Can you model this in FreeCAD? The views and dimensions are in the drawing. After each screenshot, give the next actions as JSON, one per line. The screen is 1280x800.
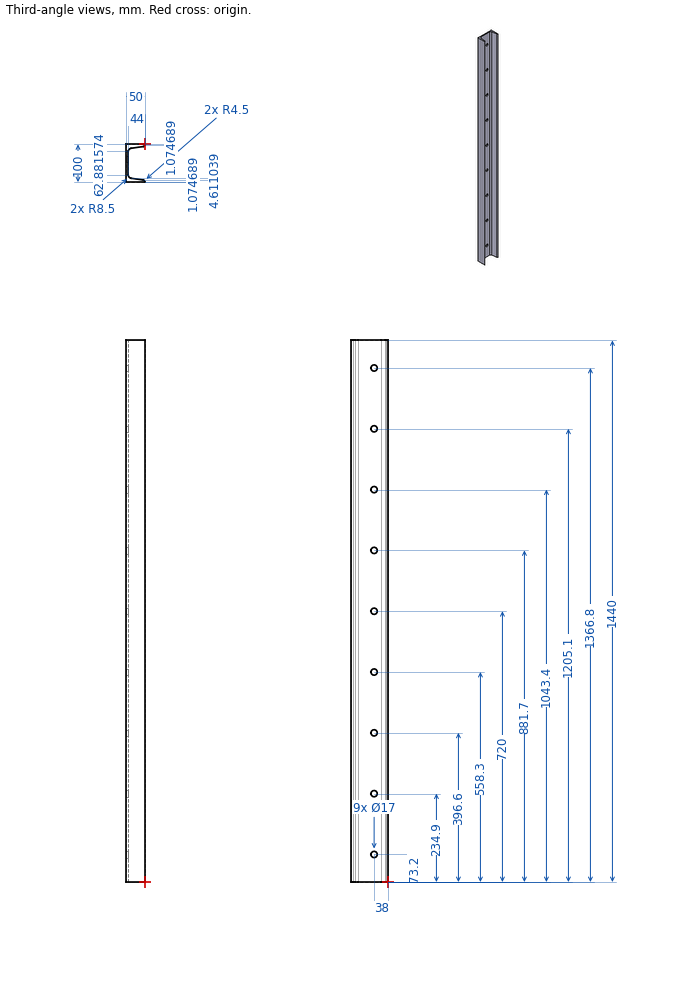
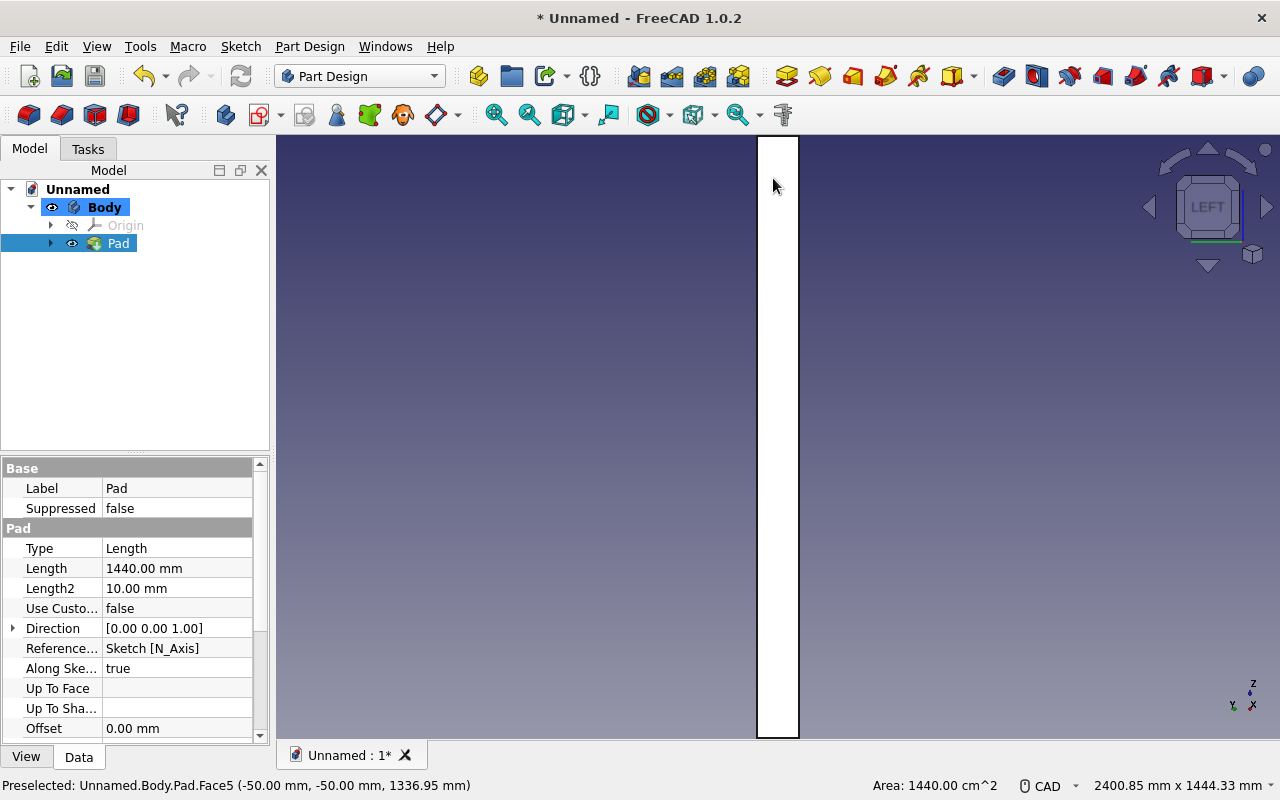
{"action": "left_click", "coordinate": [258, 116]}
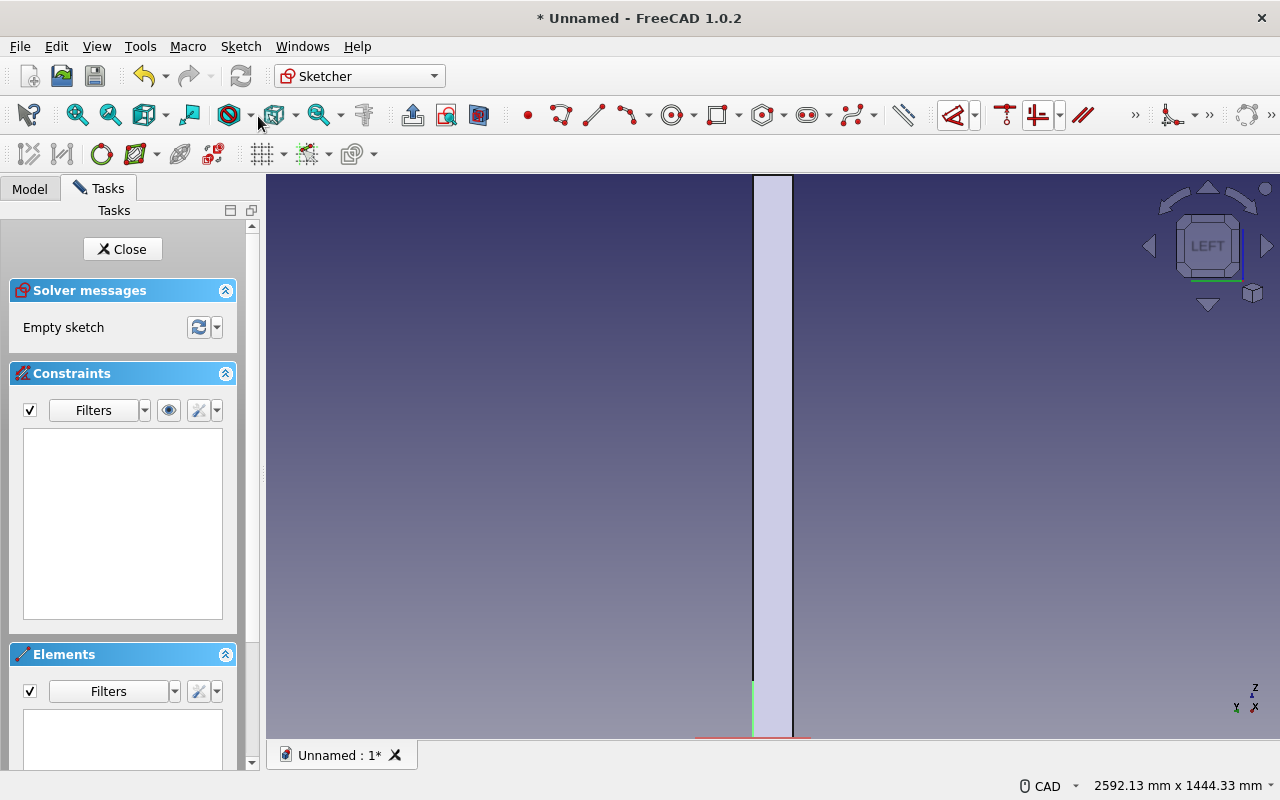
{"action": "scroll", "coordinate": [586, 431], "scroll_direction": "down", "scroll_amount": 2}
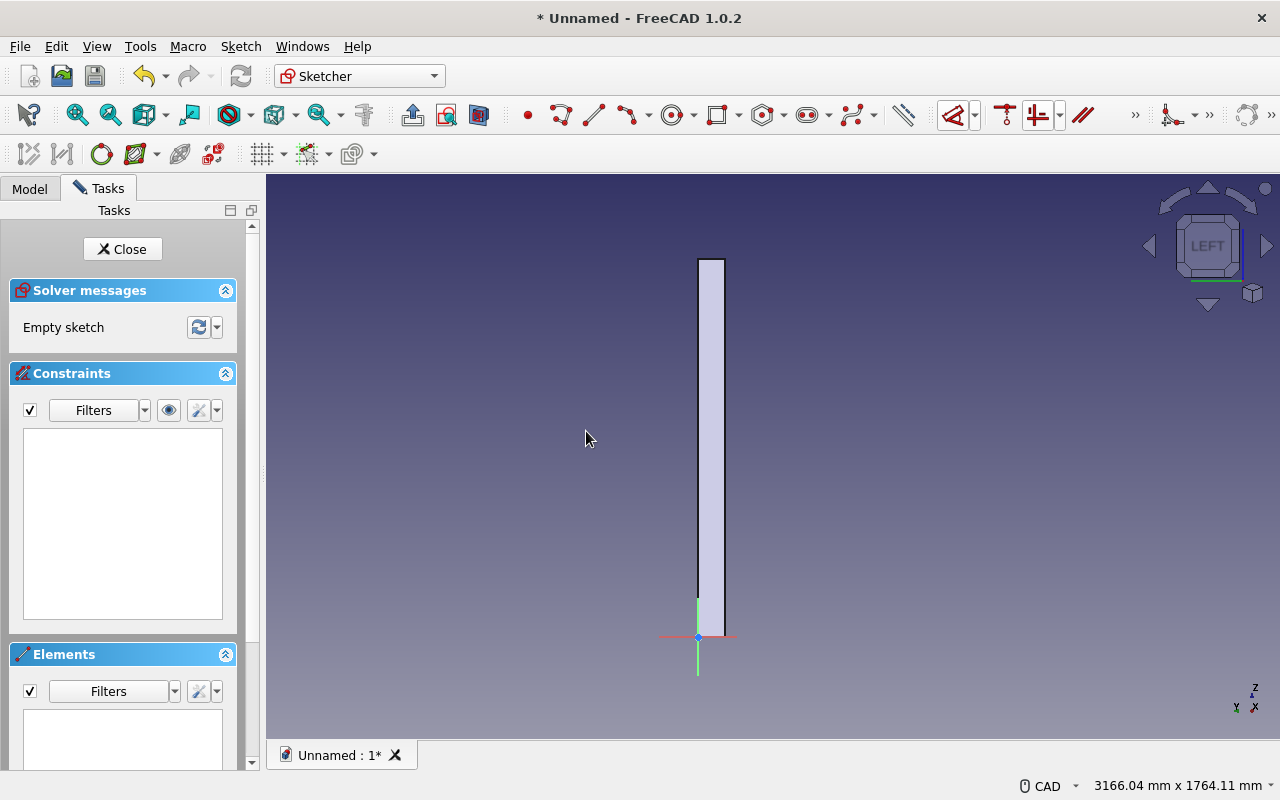
{"action": "left_click", "coordinate": [672, 116]}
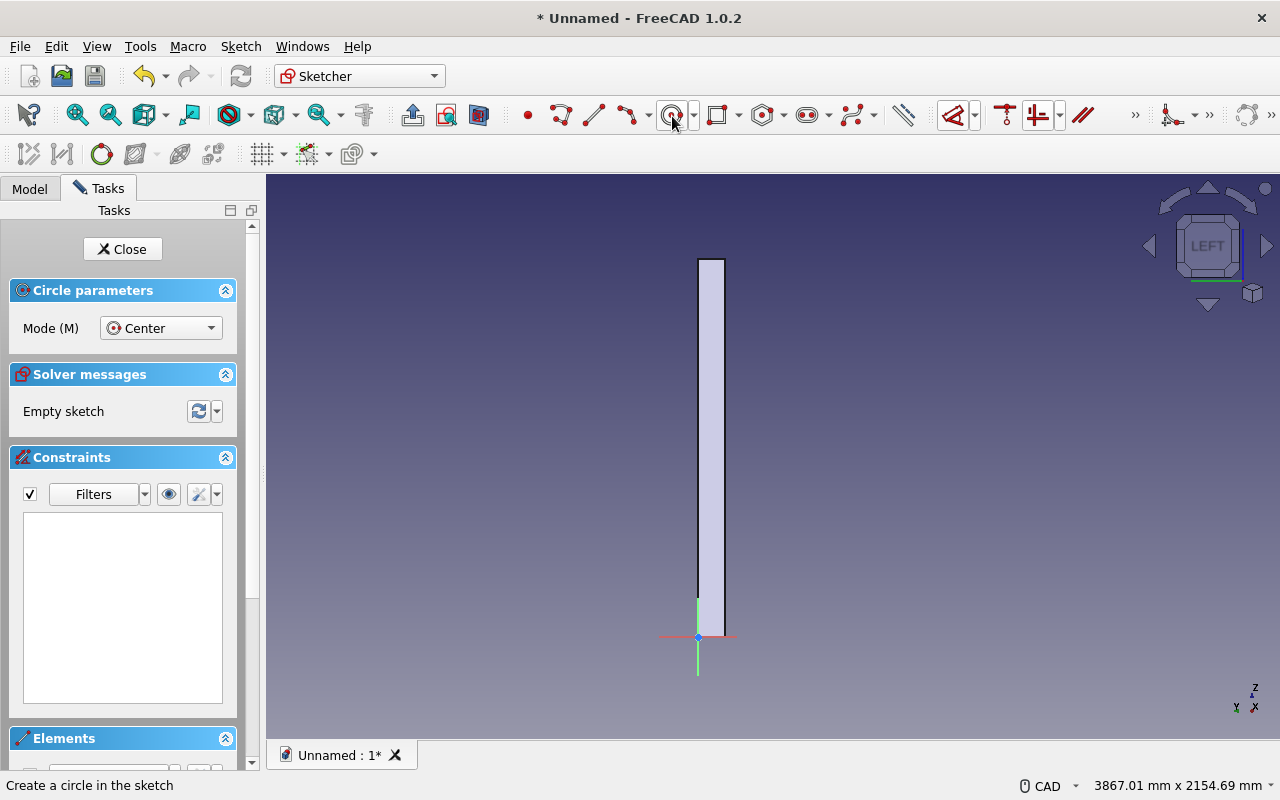
{"action": "scroll", "coordinate": [708, 618], "scroll_direction": "up", "scroll_amount": 12}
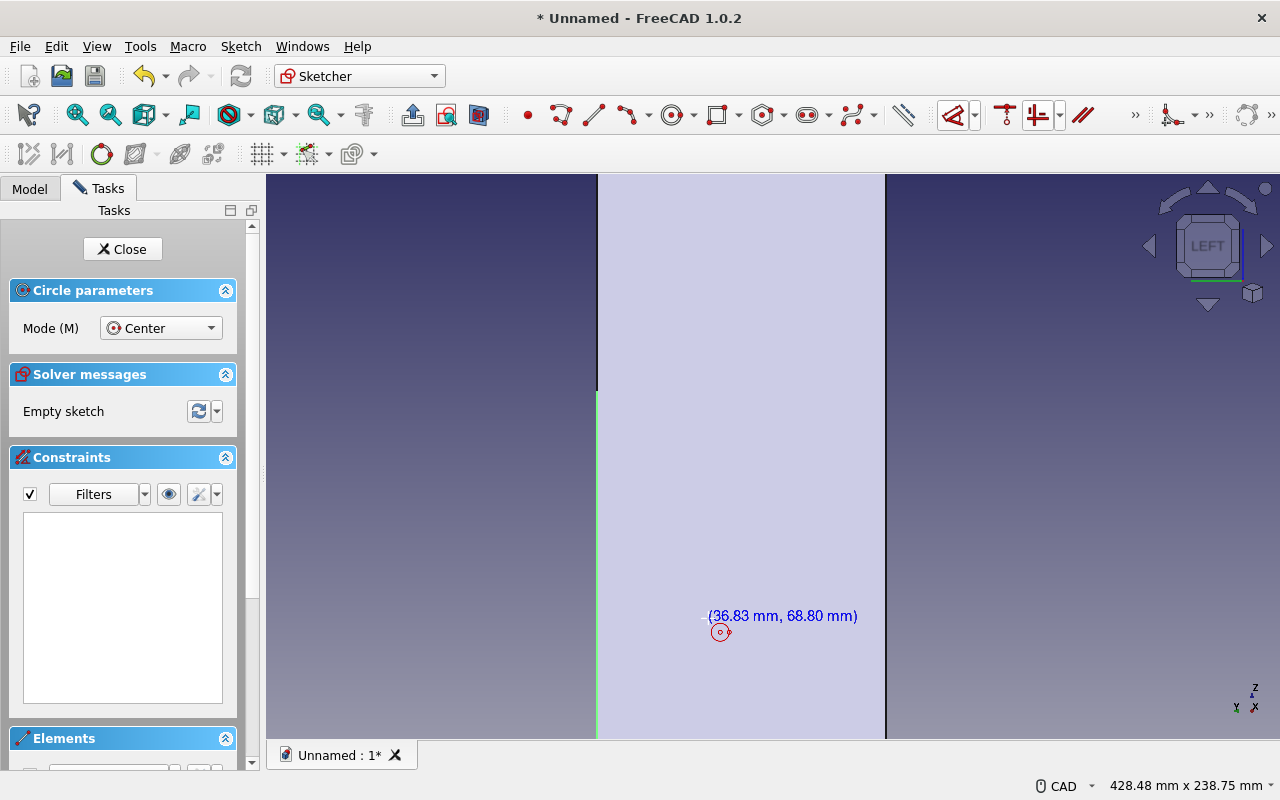
{"action": "scroll", "coordinate": [709, 619], "scroll_direction": "down", "scroll_amount": 12}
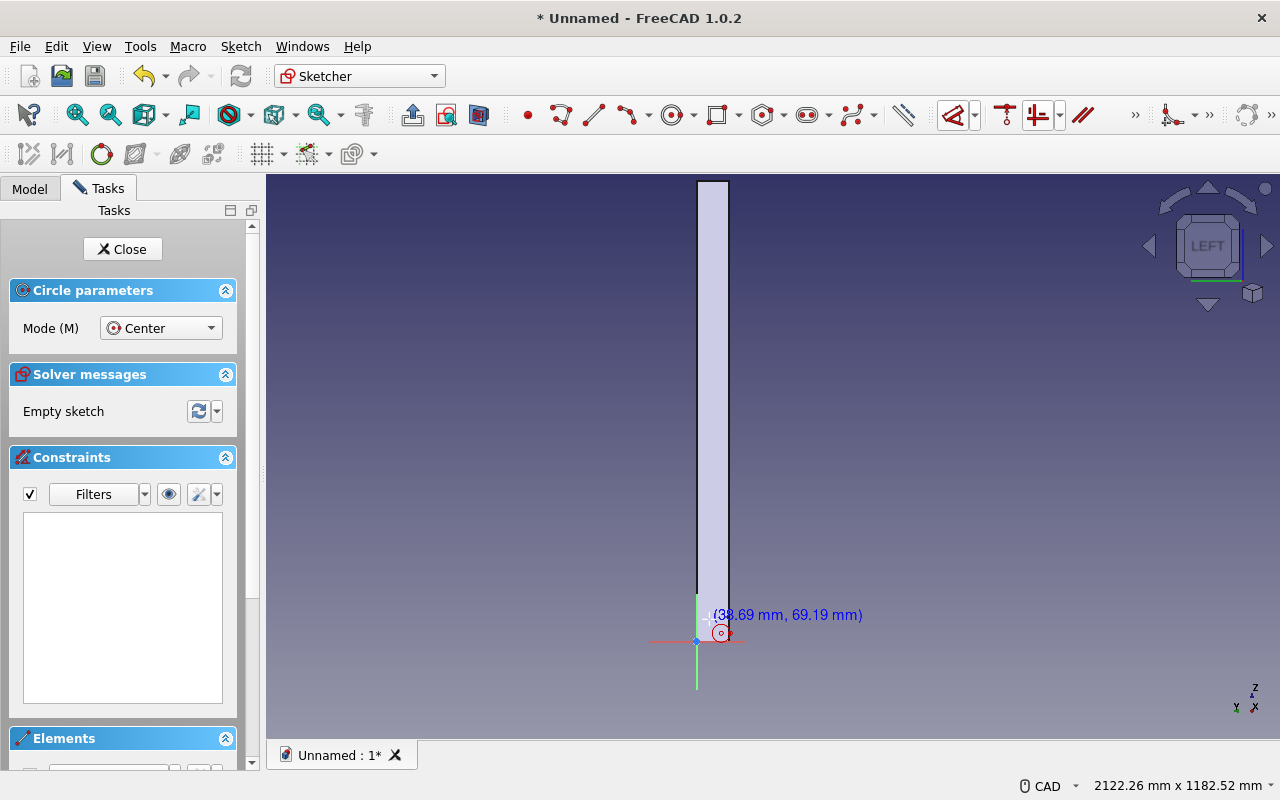
{"action": "scroll", "coordinate": [709, 619], "scroll_direction": "up", "scroll_amount": 3}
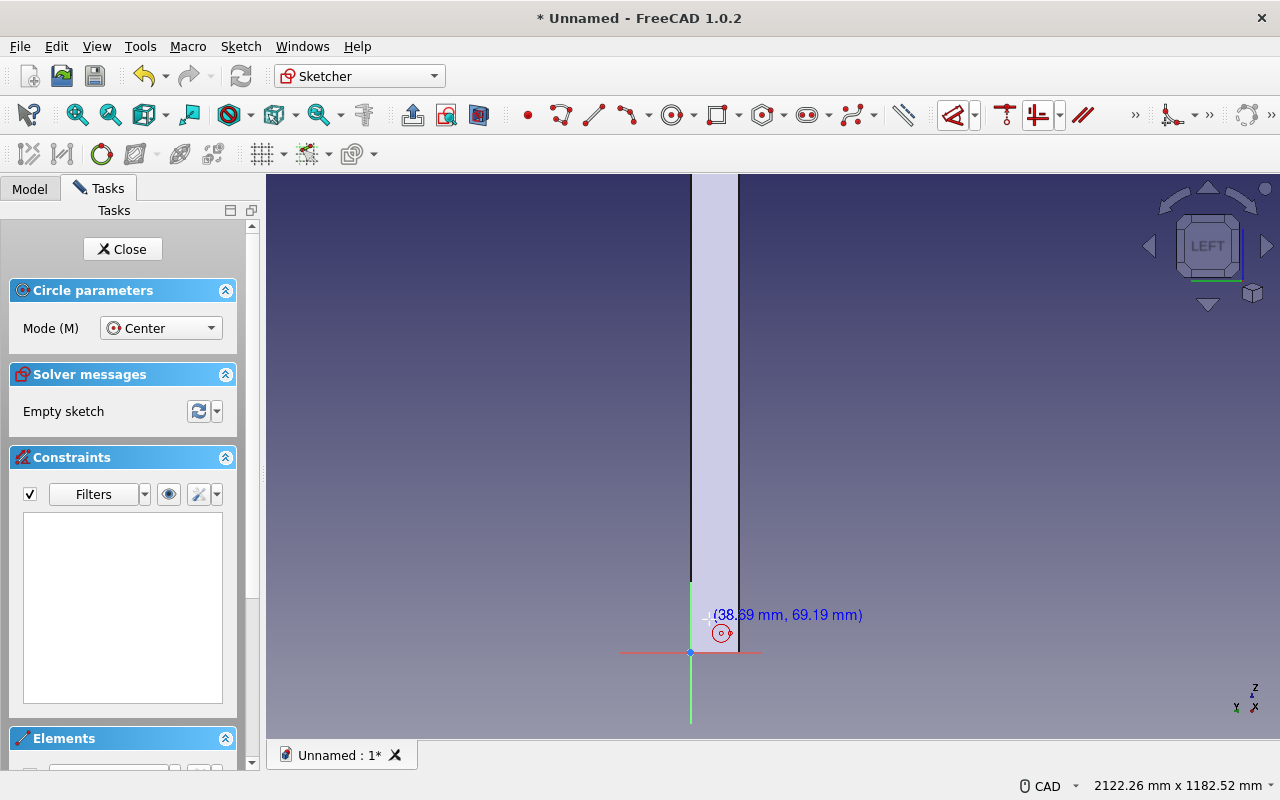
{"action": "left_click", "coordinate": [709, 618]}
{"action": "mouse_move", "coordinate": [712, 615]}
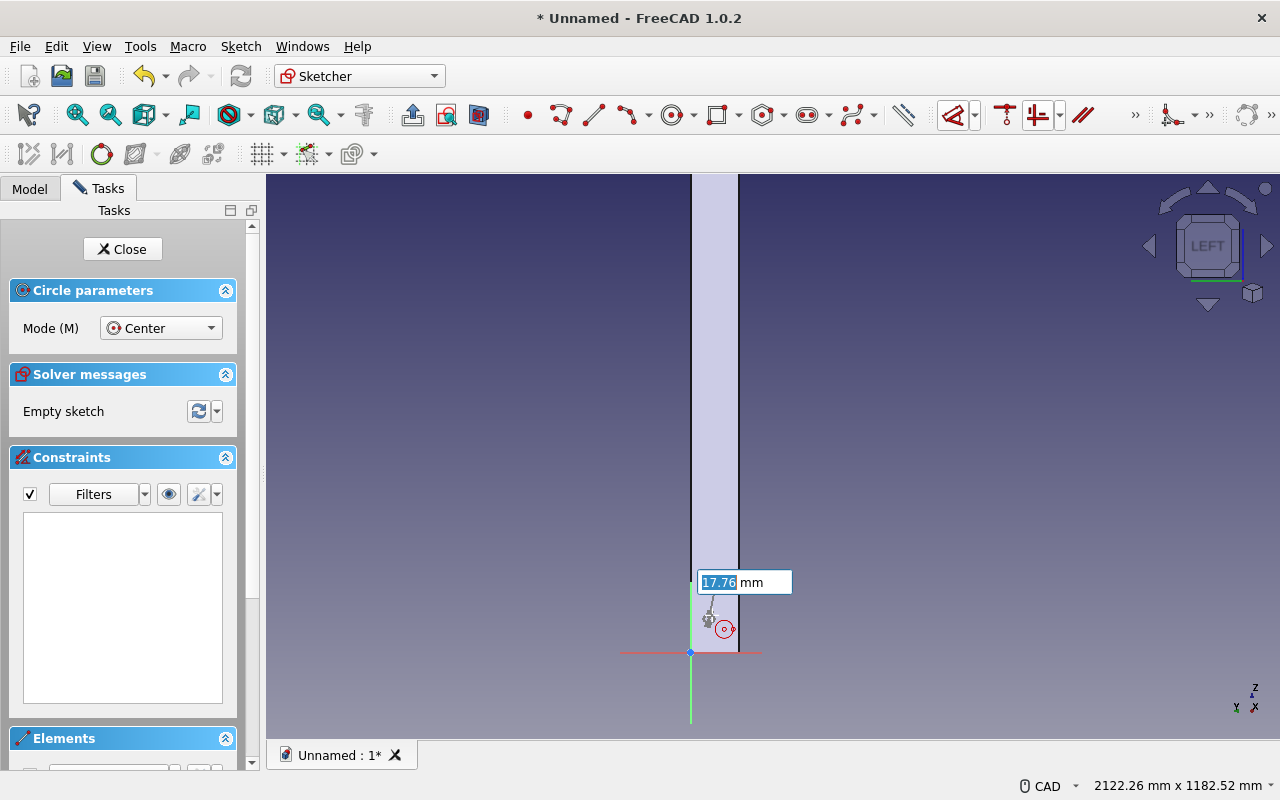
{"action": "type", "text": "17"}
{"action": "key", "text": "Return"}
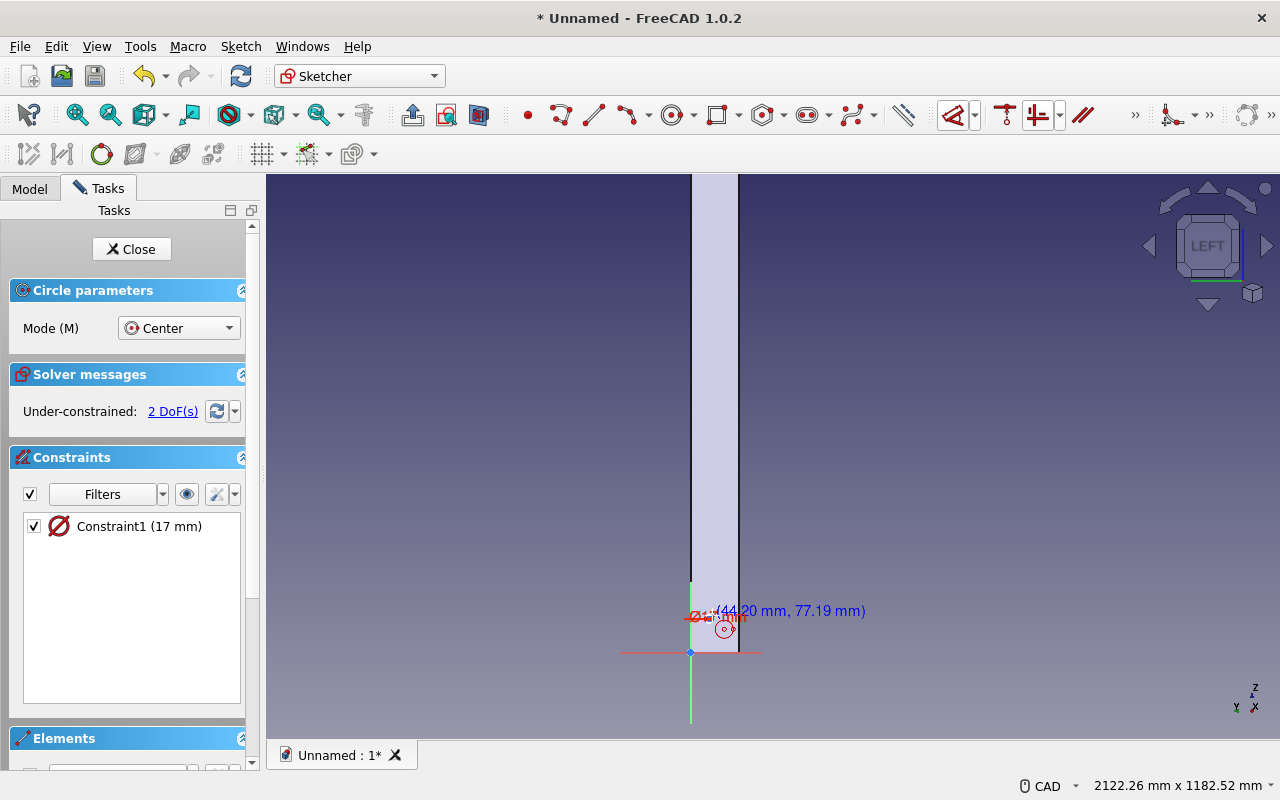
{"action": "scroll", "coordinate": [709, 541], "scroll_direction": "up", "scroll_amount": 9}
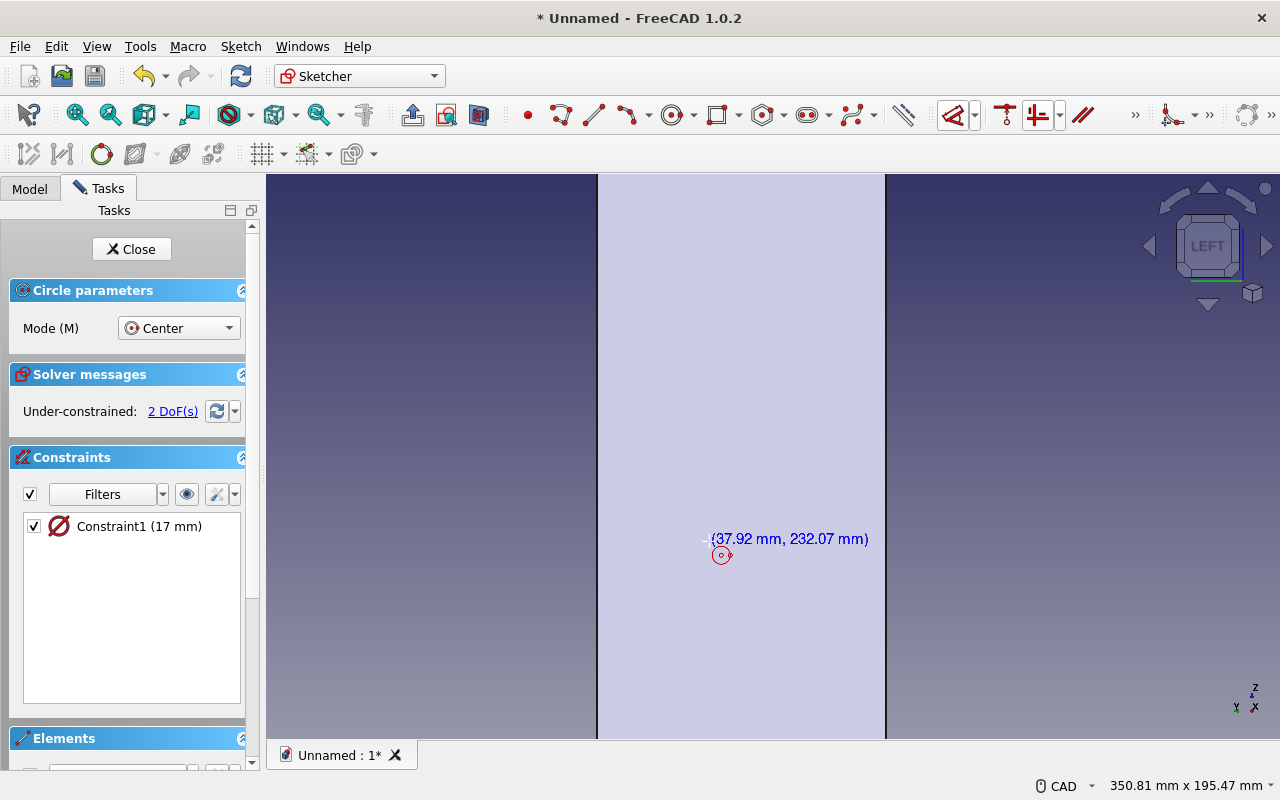
{"action": "scroll", "coordinate": [709, 579], "scroll_direction": "down", "scroll_amount": 12}